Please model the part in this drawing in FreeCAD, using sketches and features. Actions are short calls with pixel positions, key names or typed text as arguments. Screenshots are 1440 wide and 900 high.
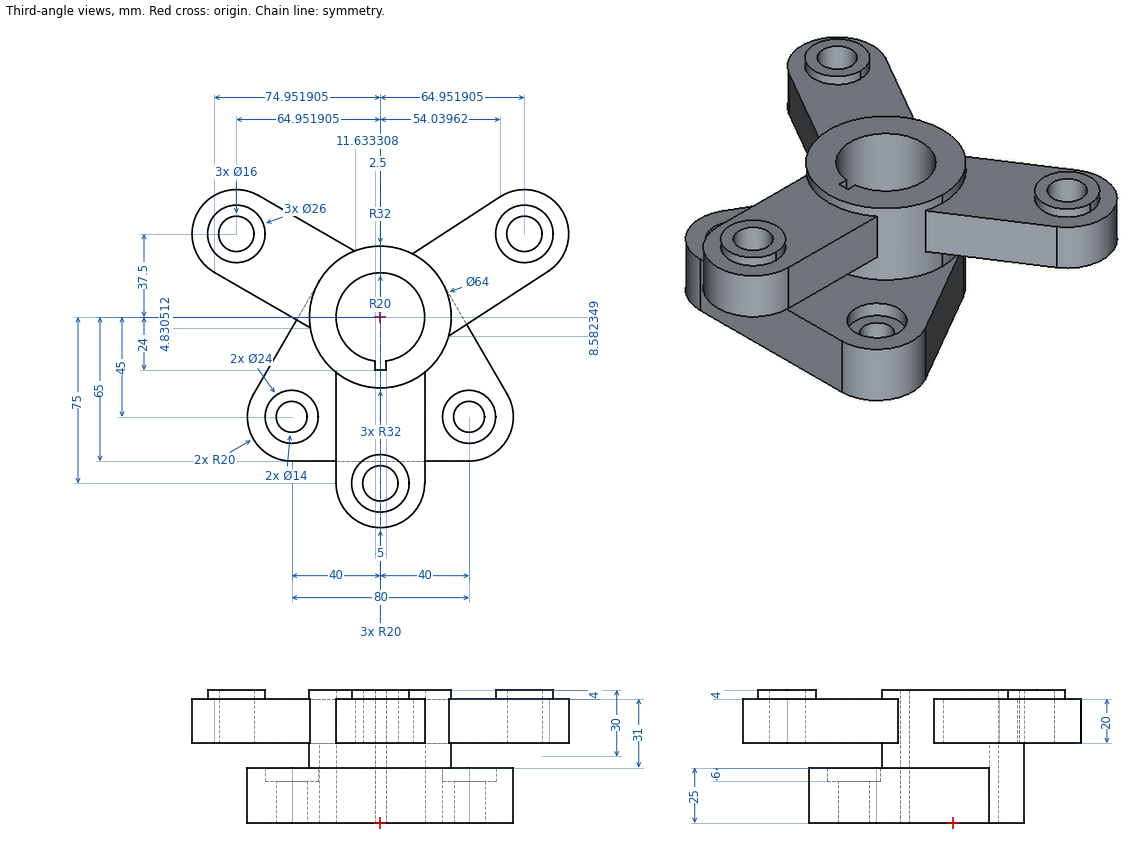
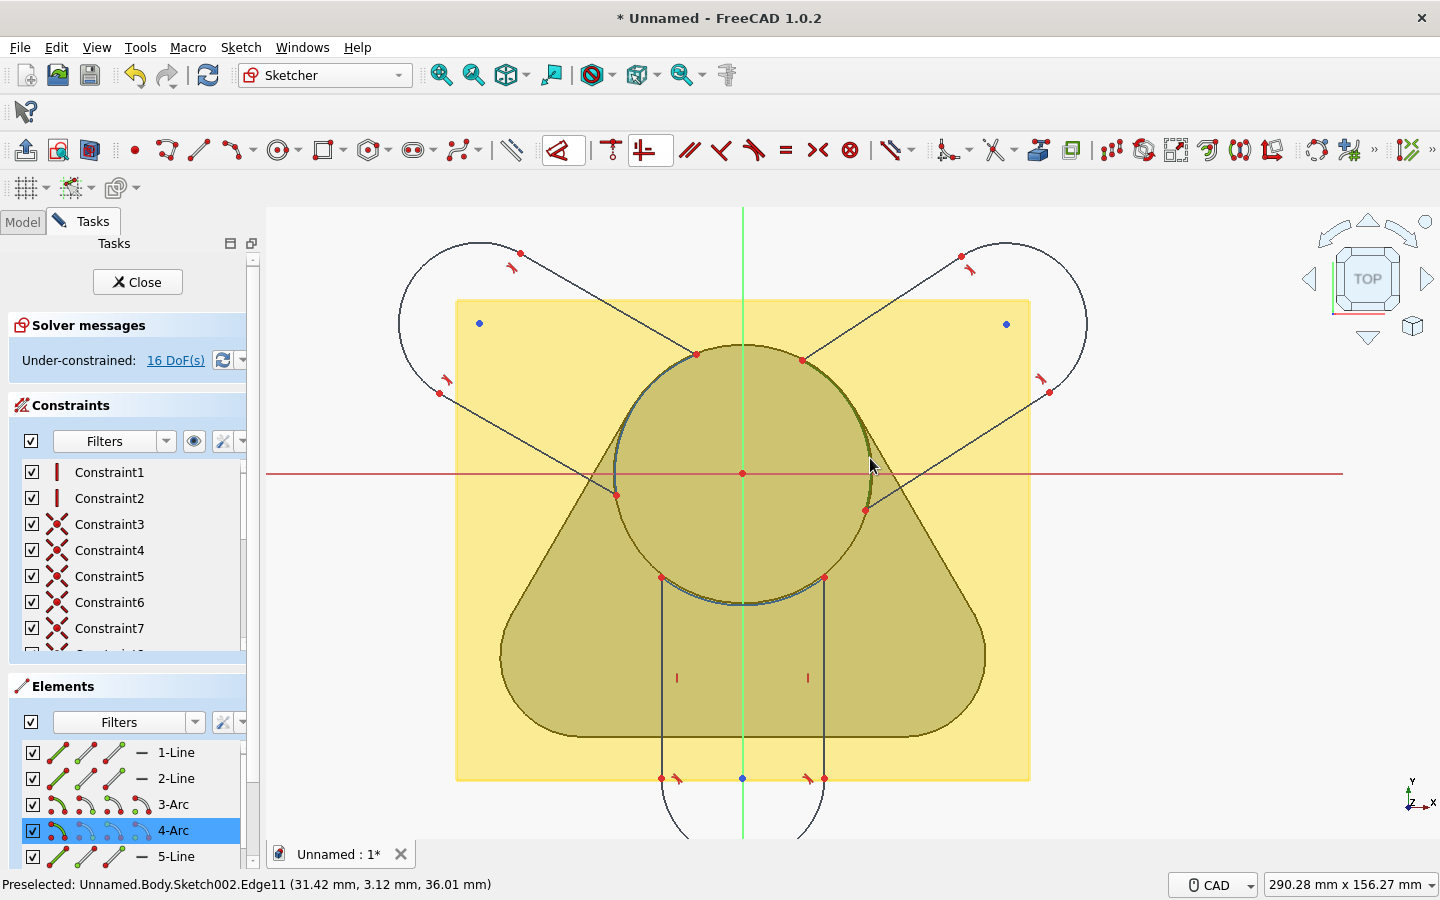
click(786, 150)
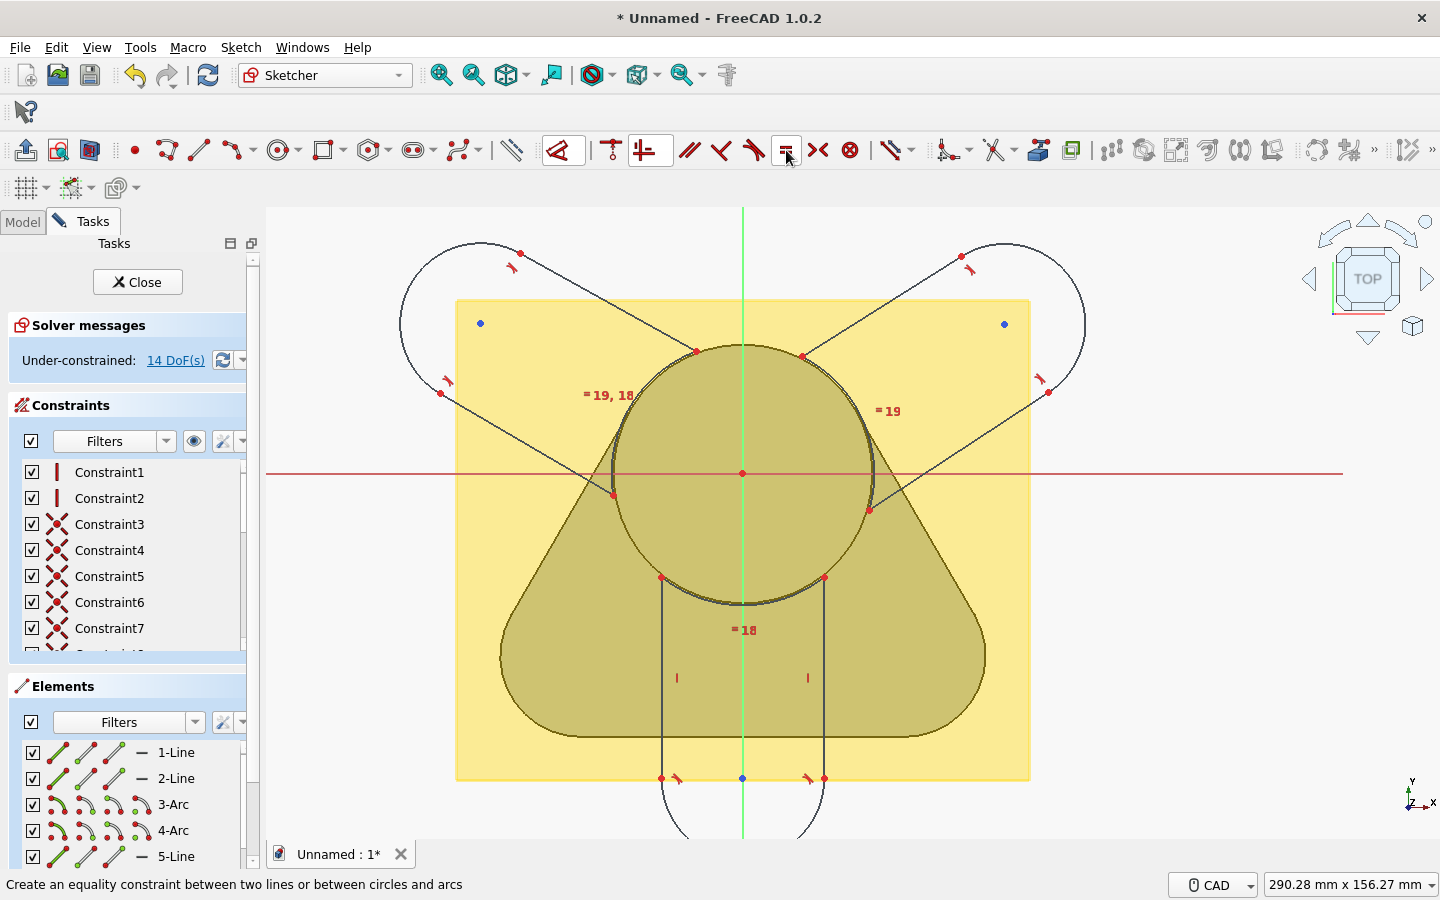
scroll(871, 457, down, 2)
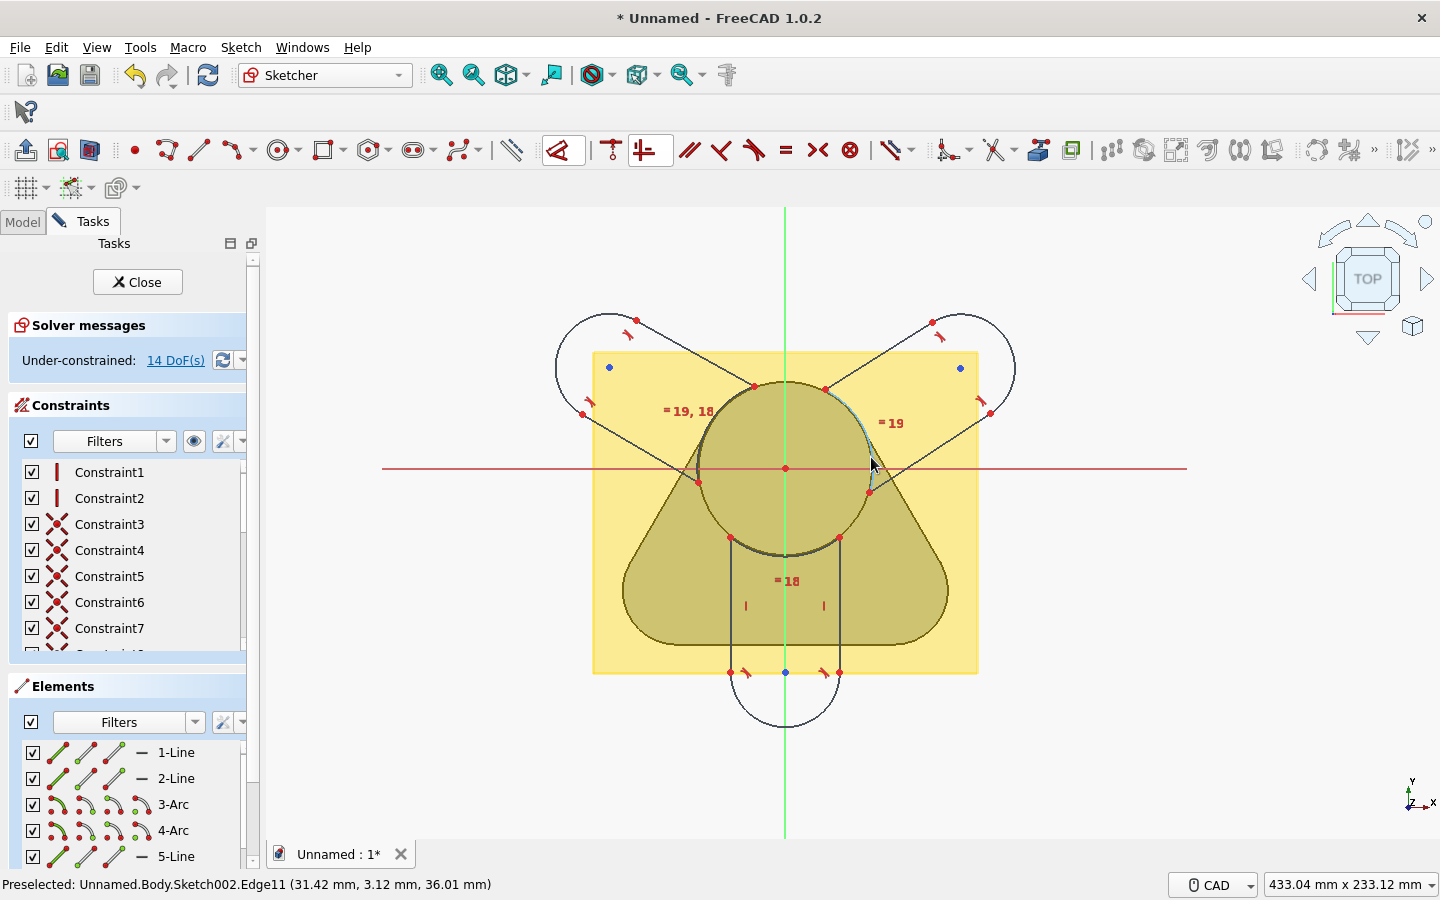
click(753, 717)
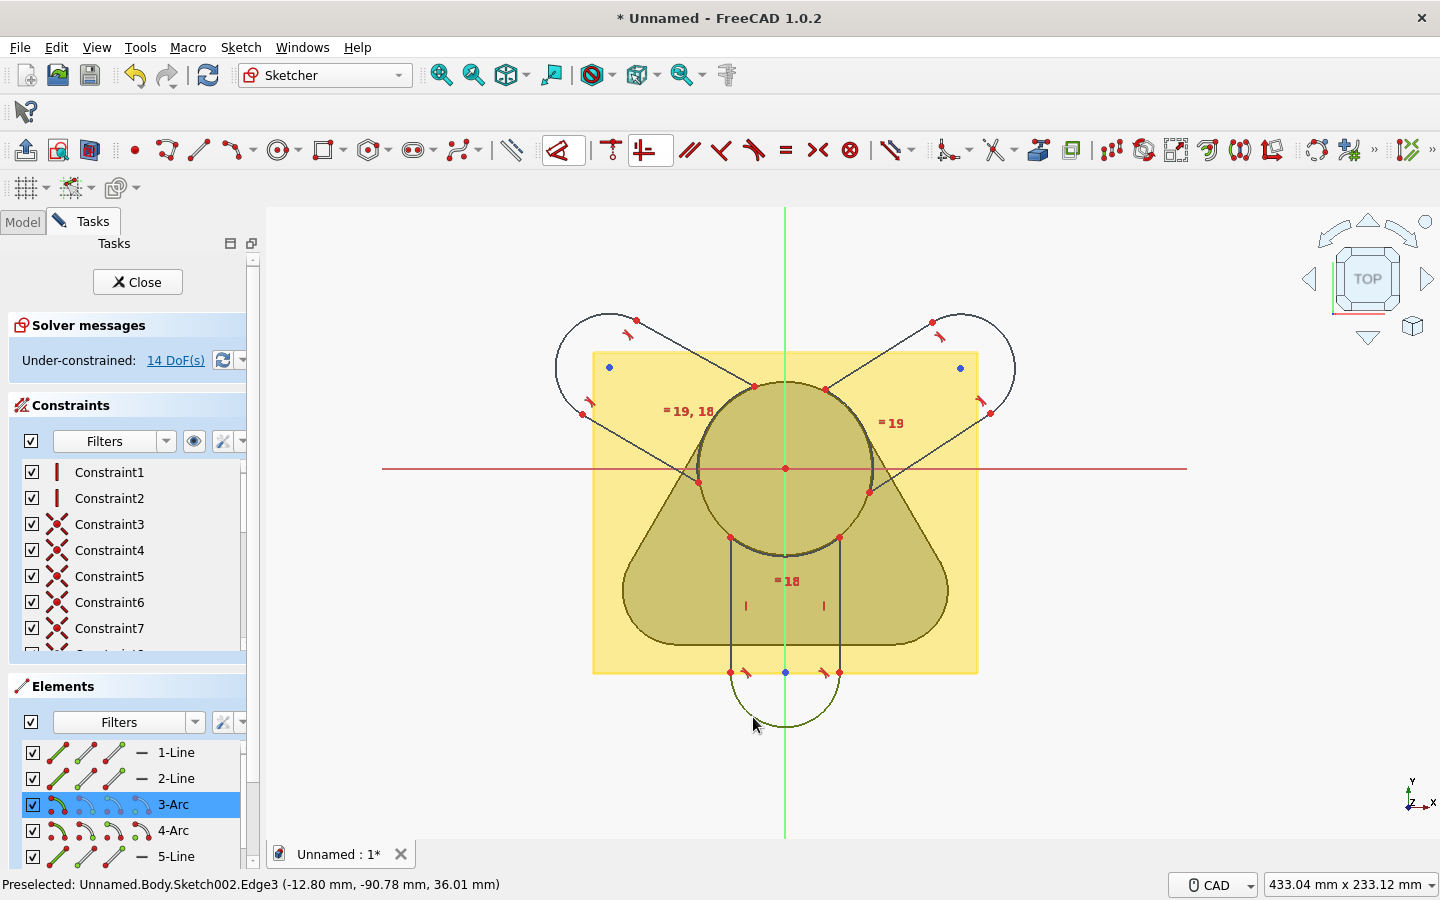
click(587, 319)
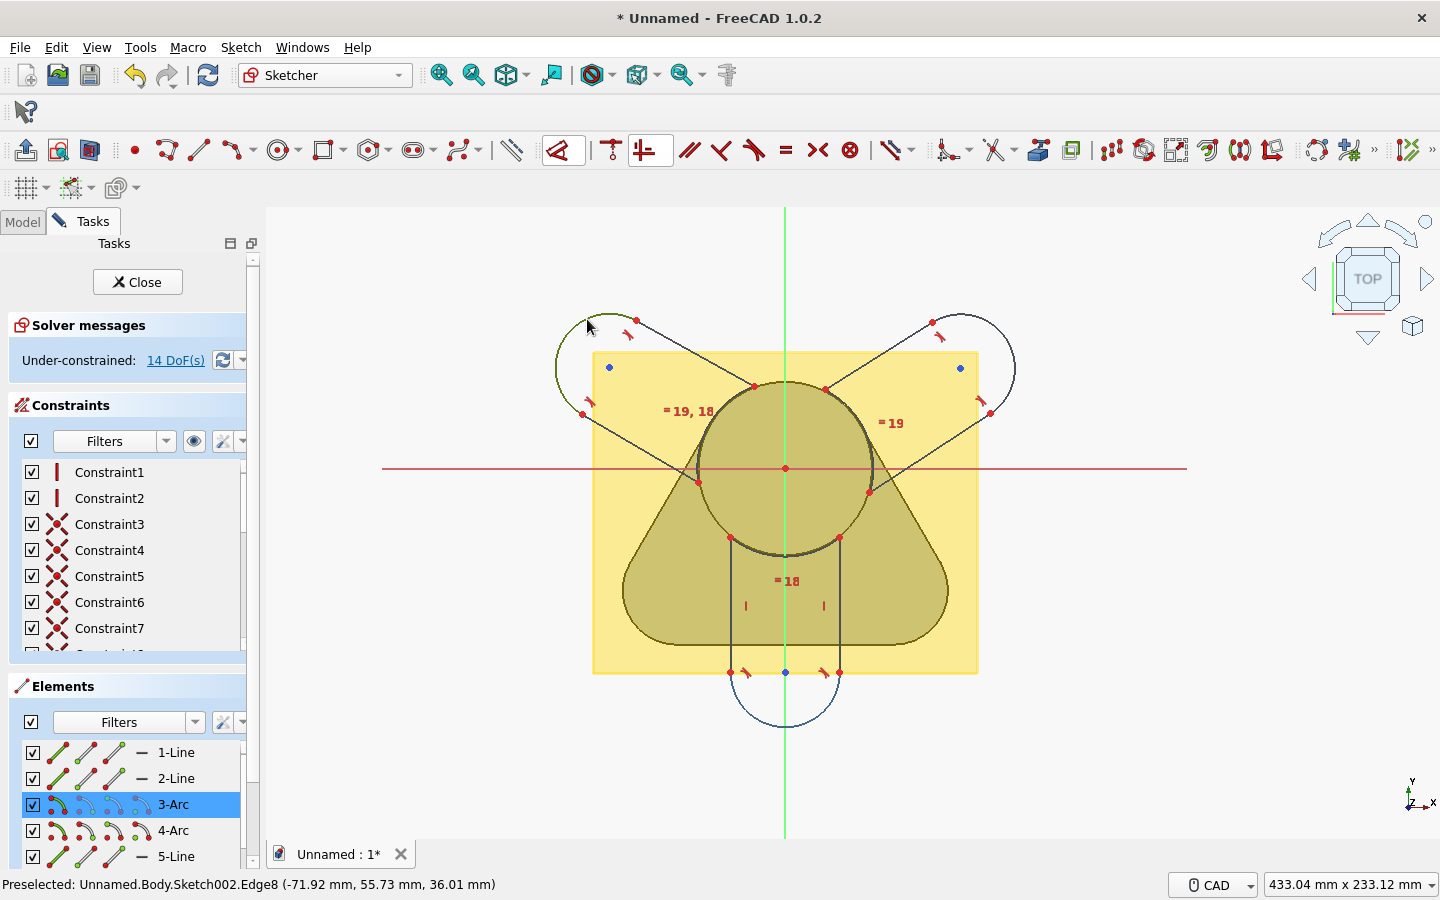
click(1015, 371)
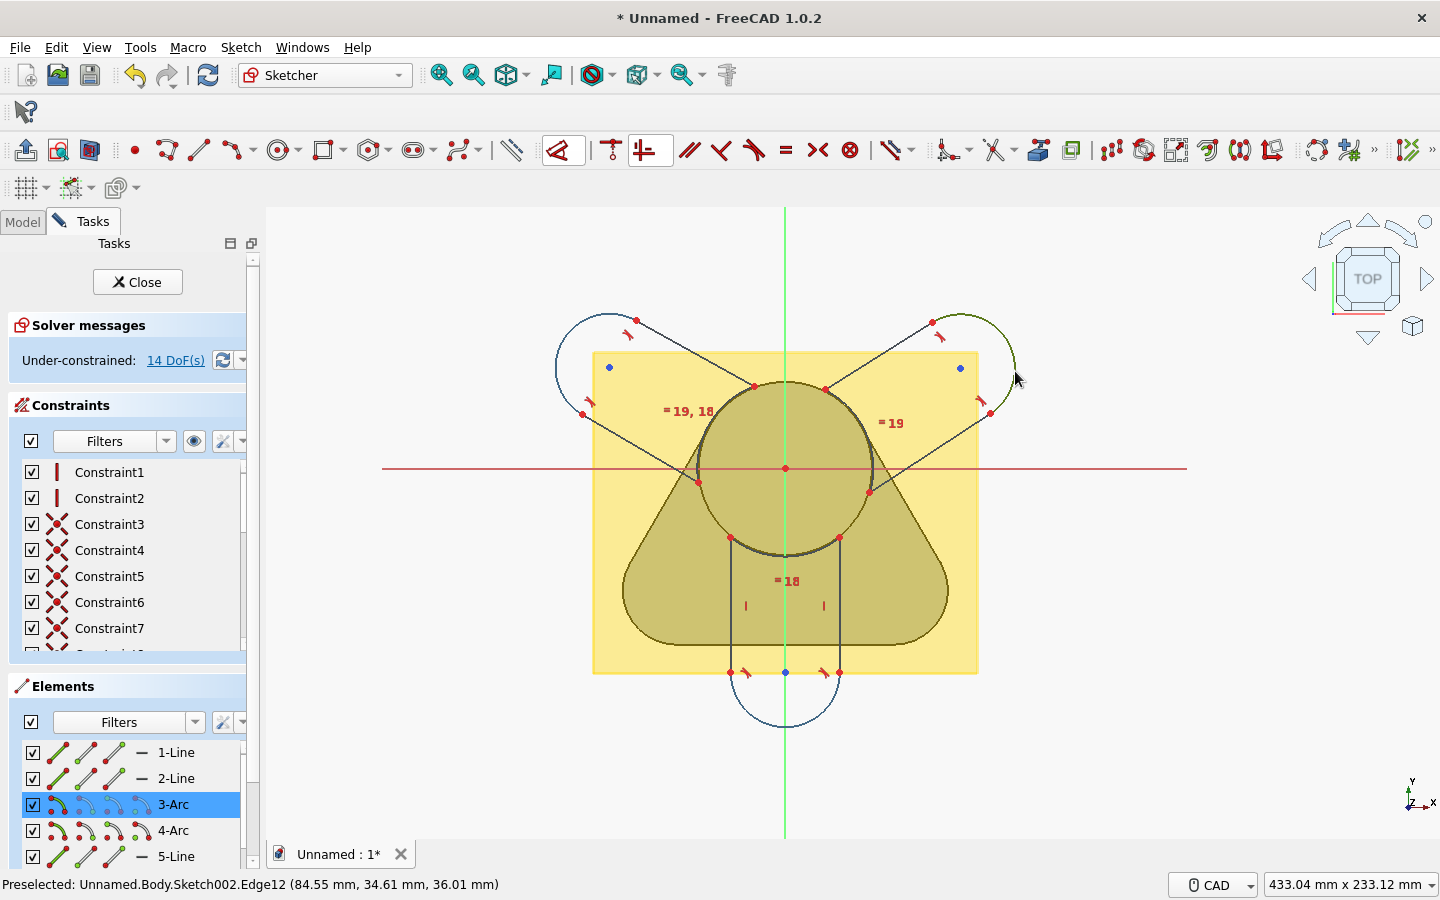
key(e)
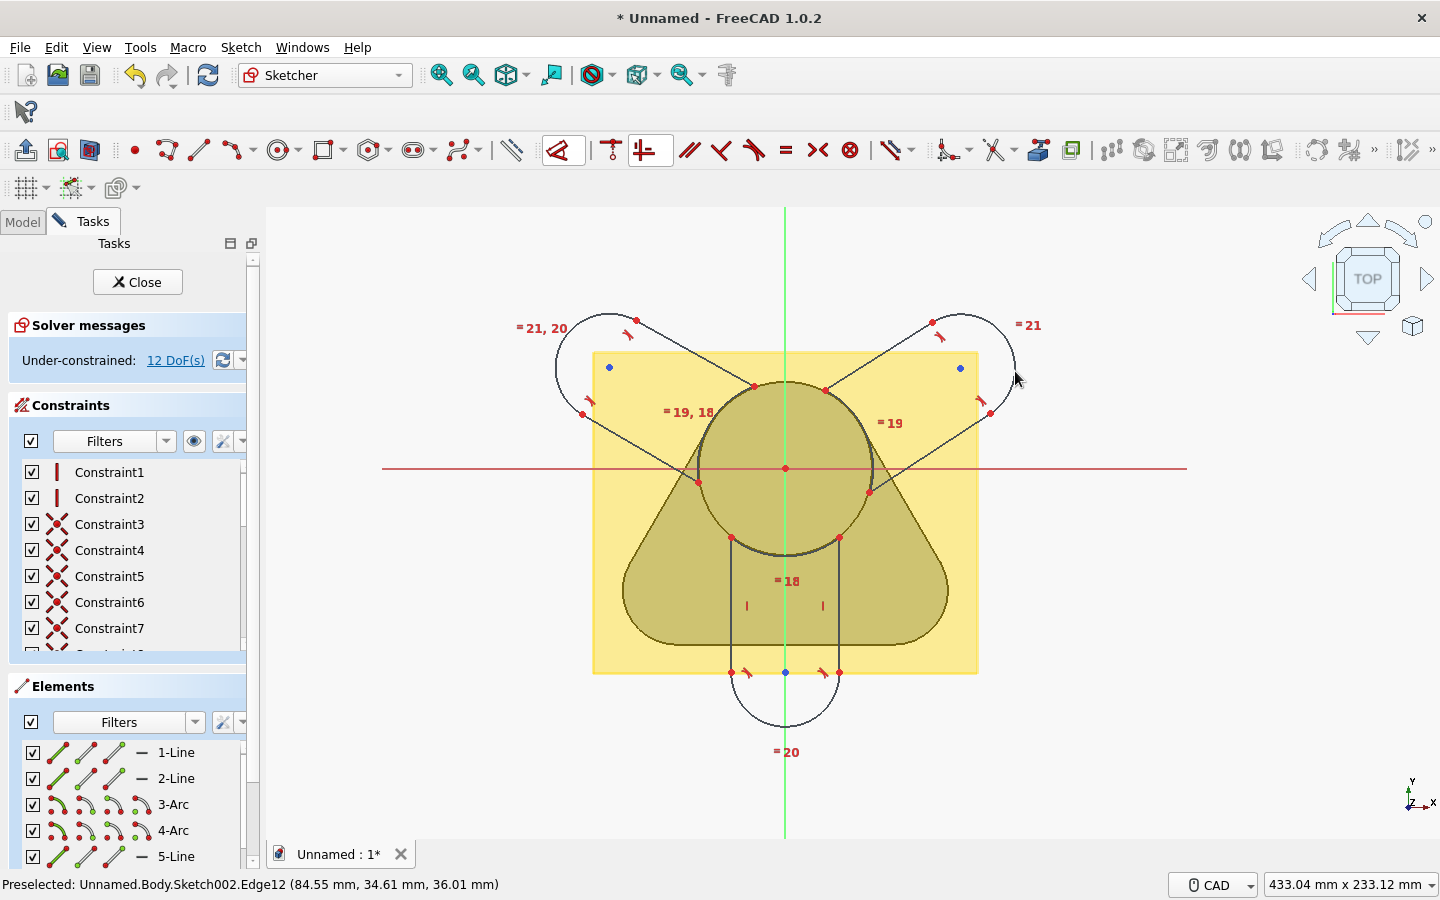
click(785, 673)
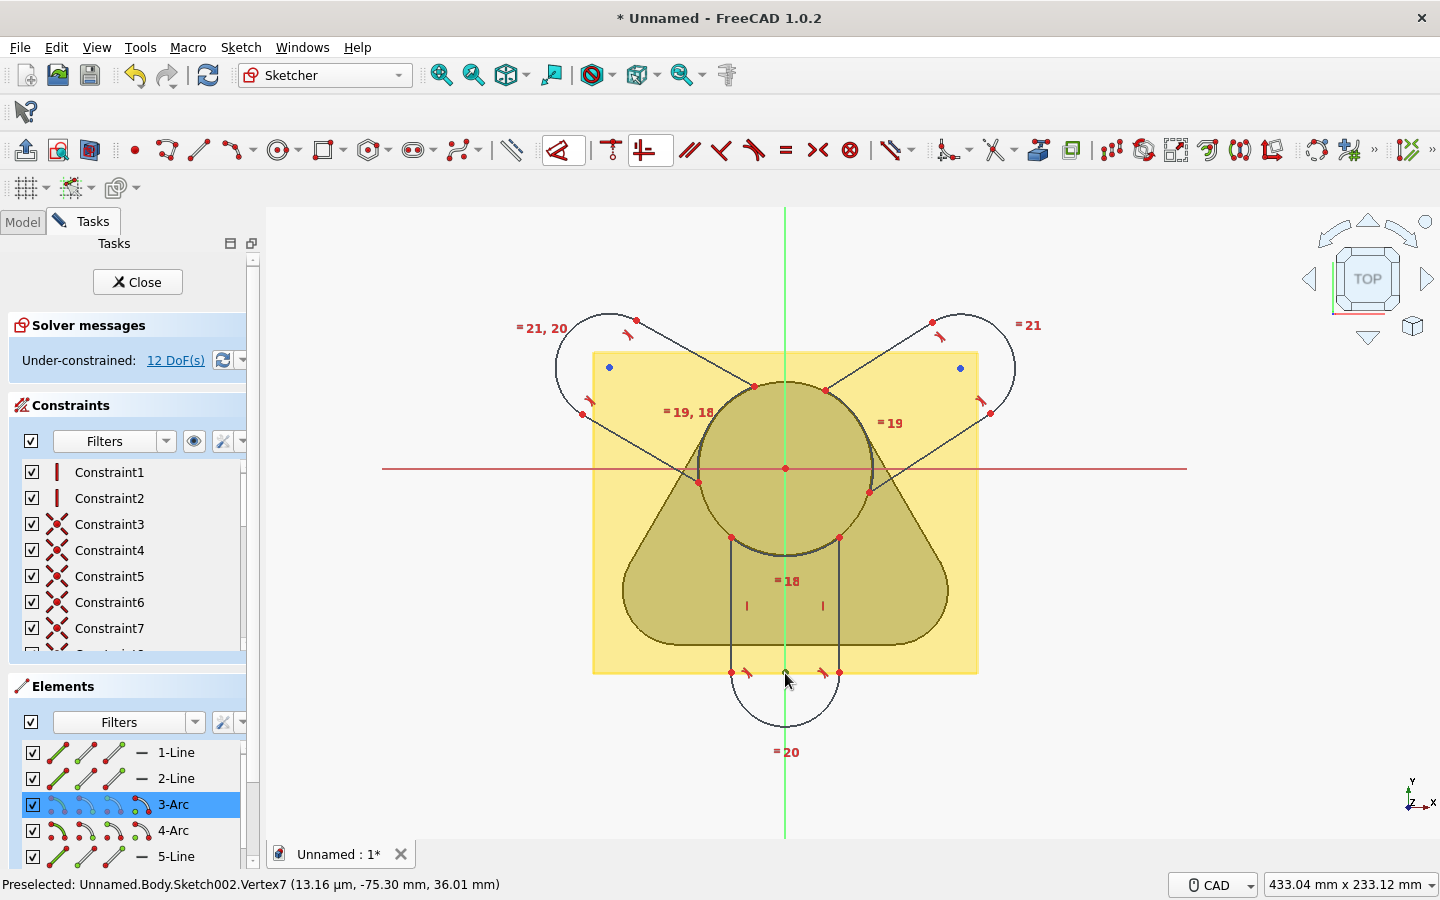
click(785, 770)